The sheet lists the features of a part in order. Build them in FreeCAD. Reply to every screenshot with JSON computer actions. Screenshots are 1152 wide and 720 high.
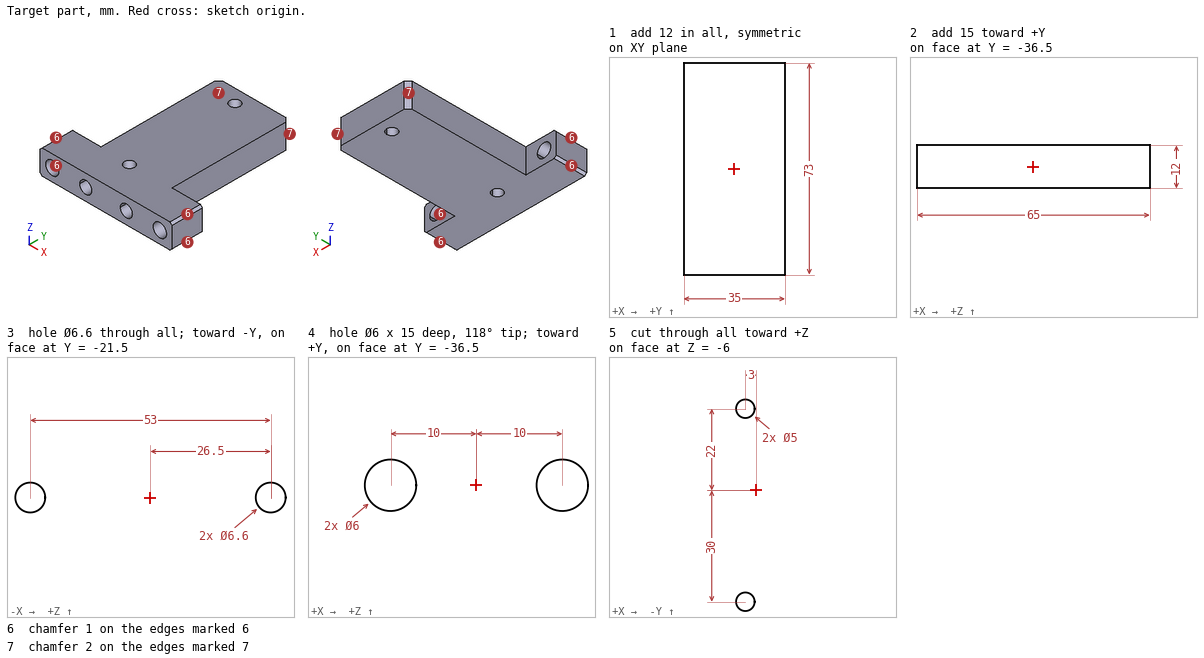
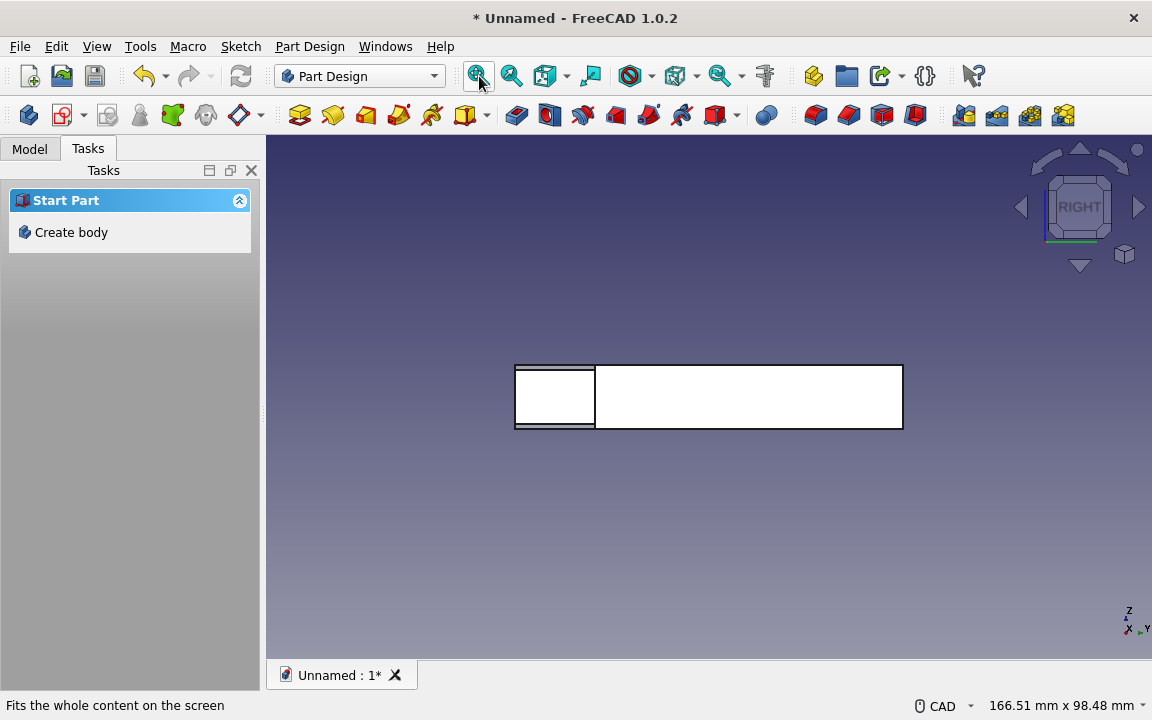
{"action": "left_click", "coordinate": [903, 396]}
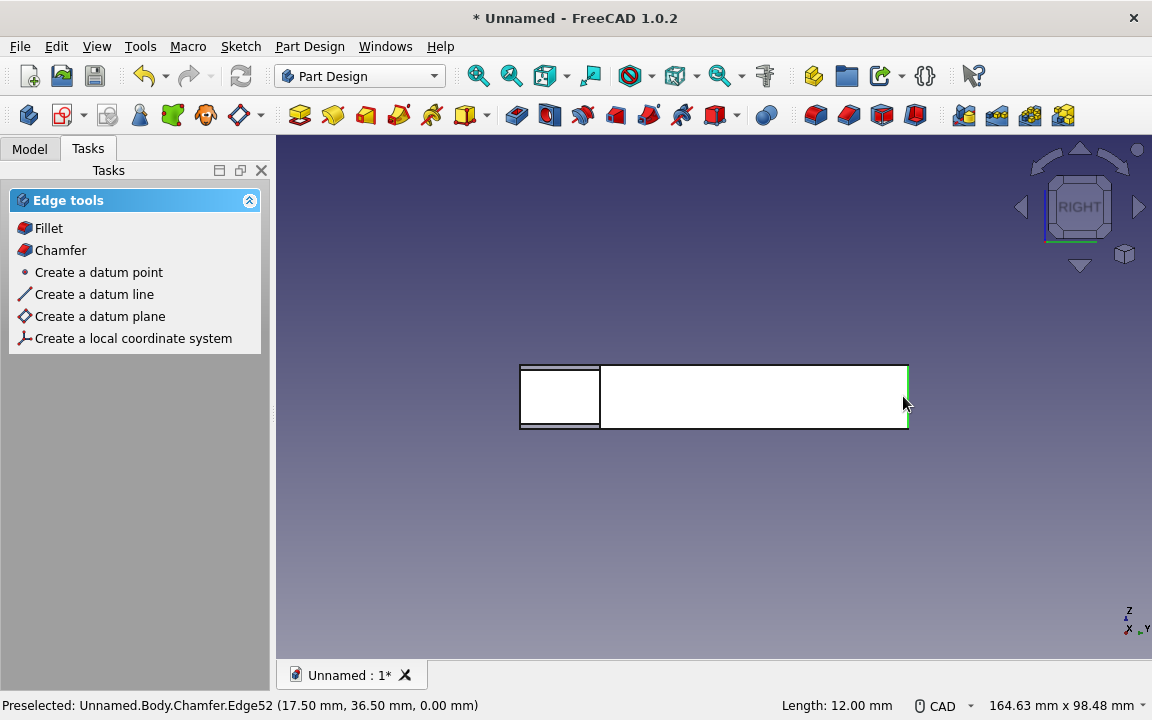
{"action": "key", "text": "5"}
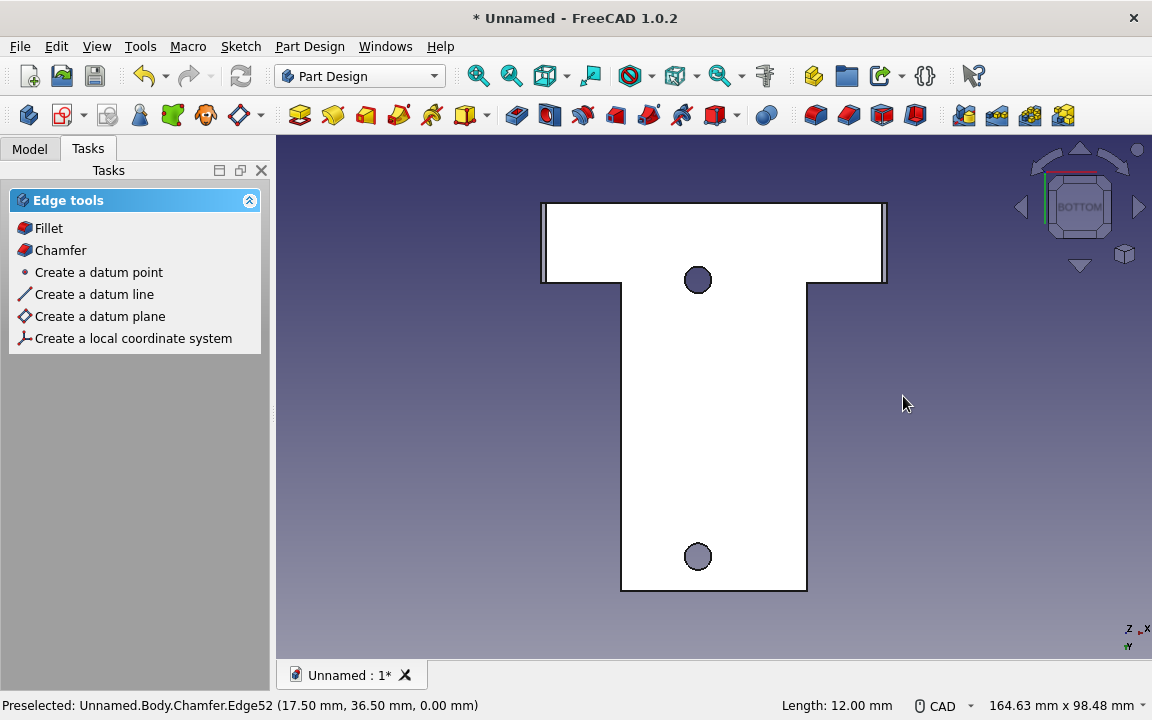
{"action": "key", "text": "4"}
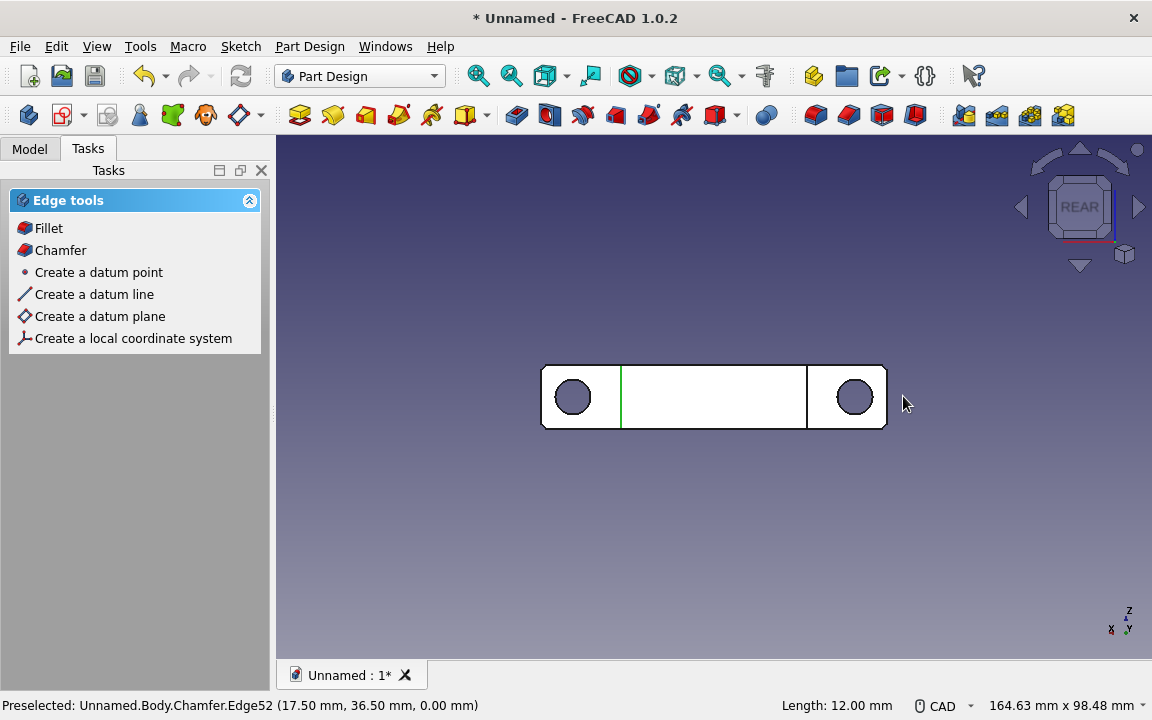
{"action": "left_click", "coordinate": [479, 76]}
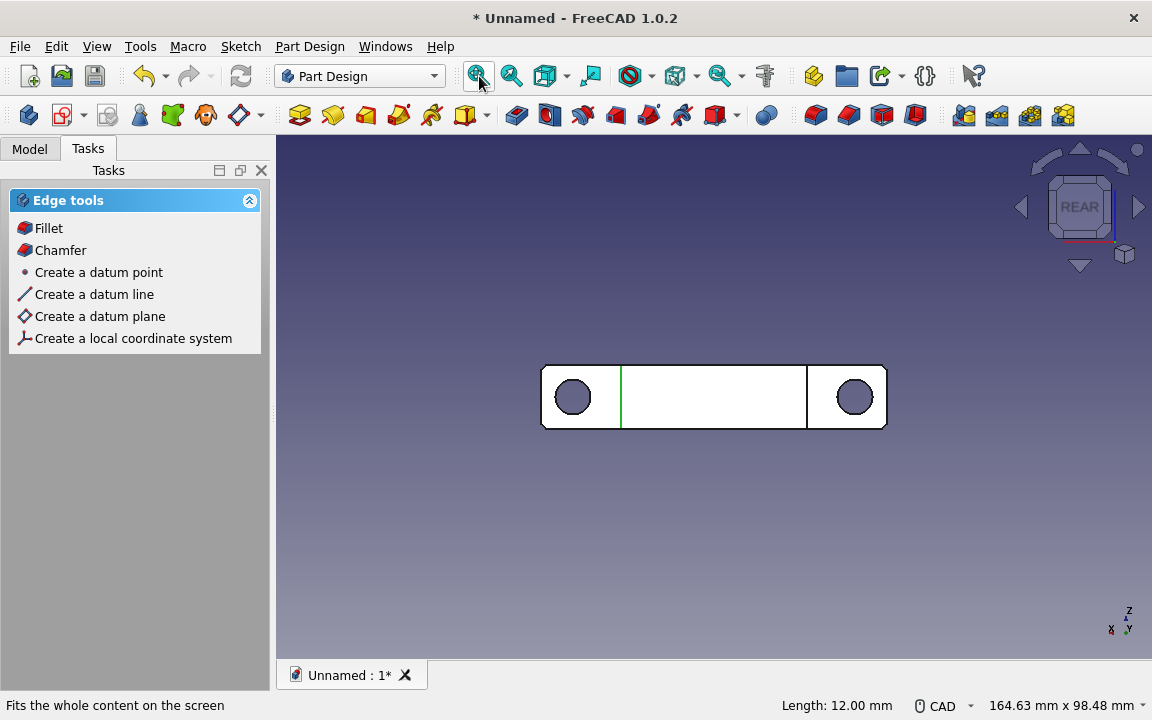
{"action": "left_click", "coordinate": [807, 396], "text": "ctrl"}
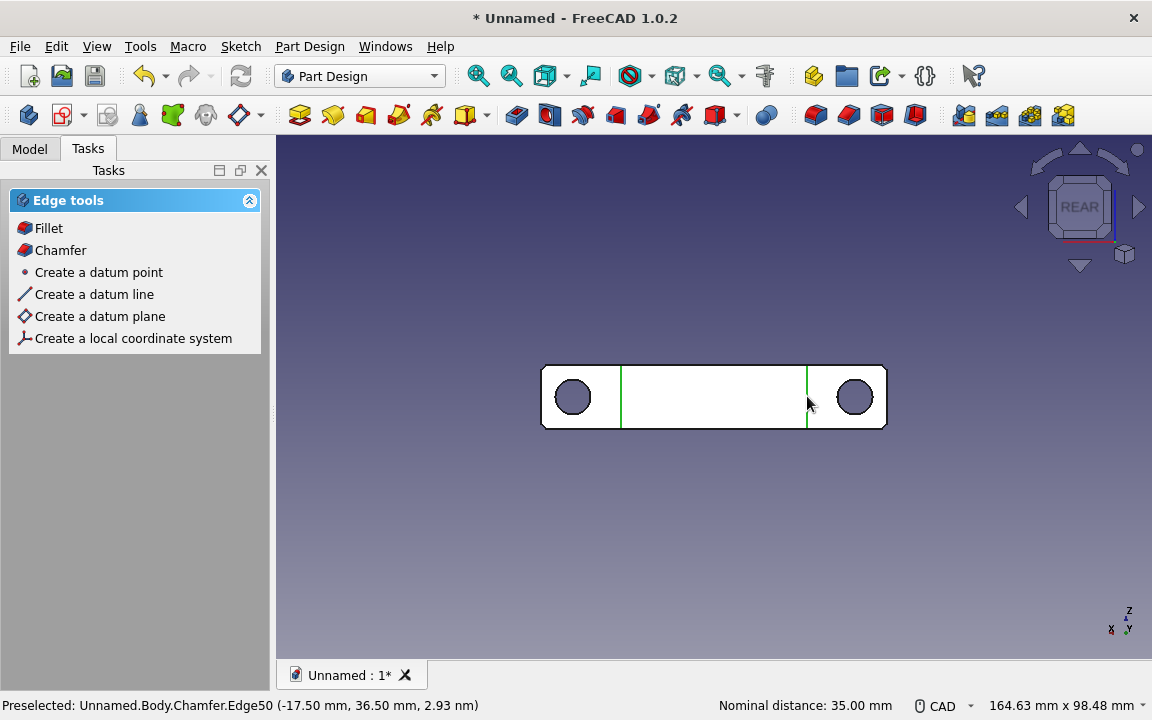
{"action": "left_click", "coordinate": [849, 116]}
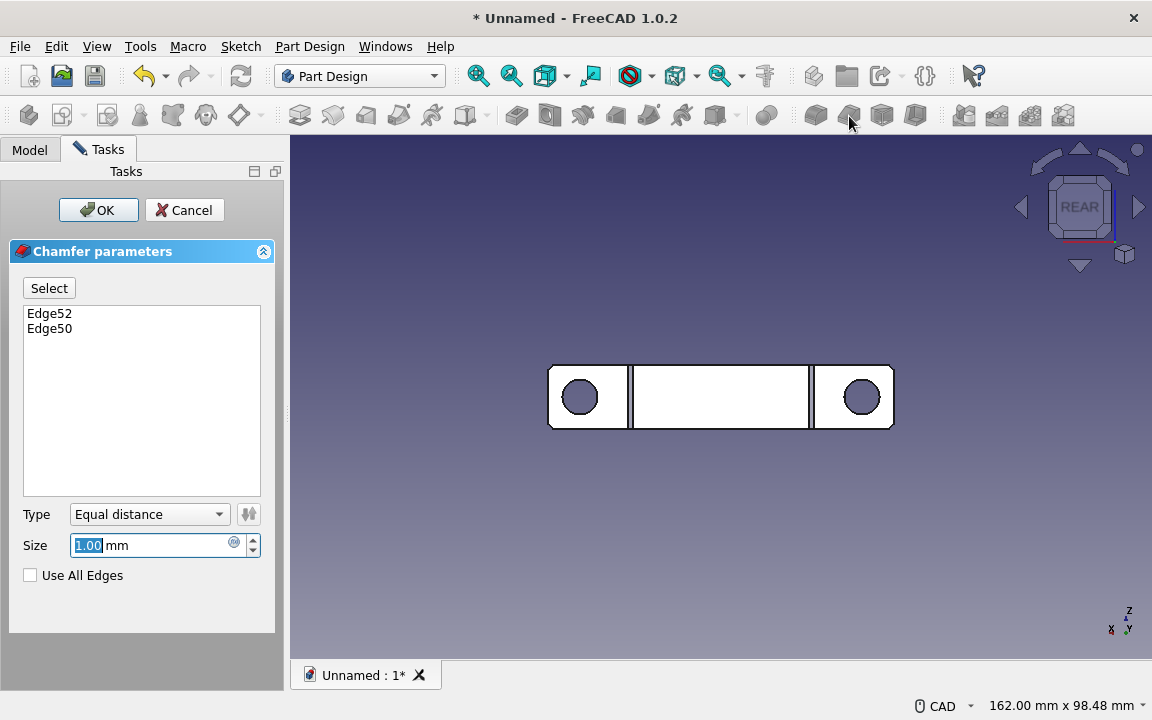
{"action": "type", "text": "2"}
{"action": "key", "text": "Tab"}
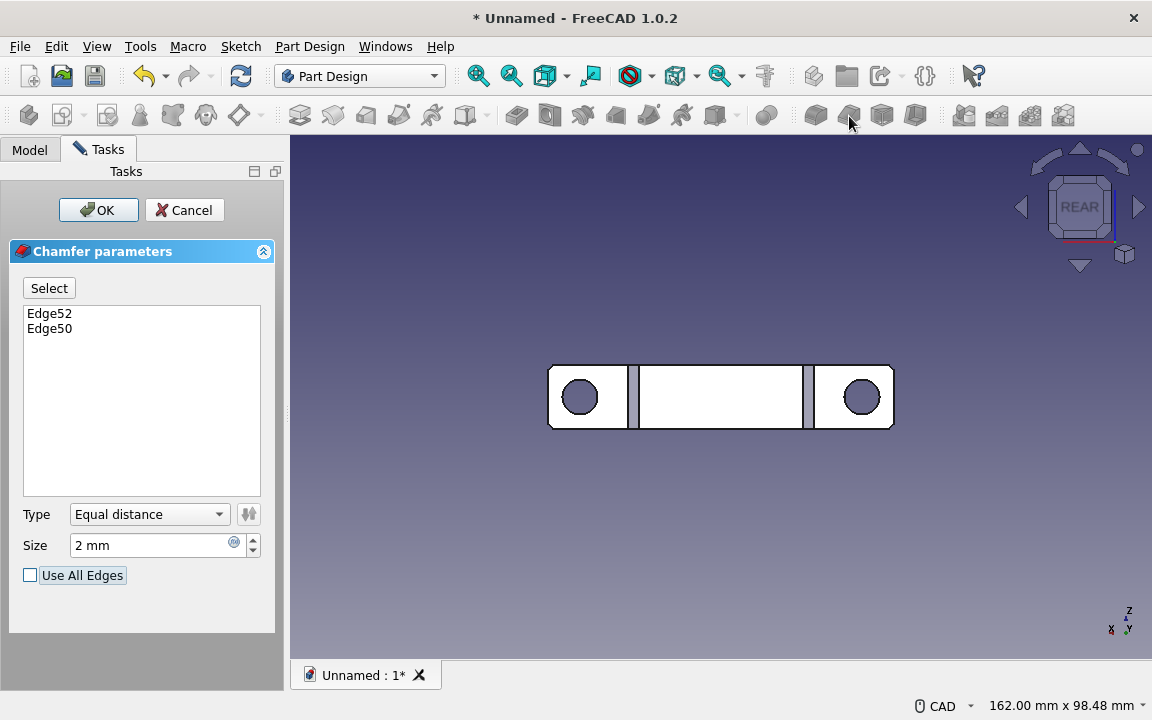
{"action": "left_click", "coordinate": [99, 210]}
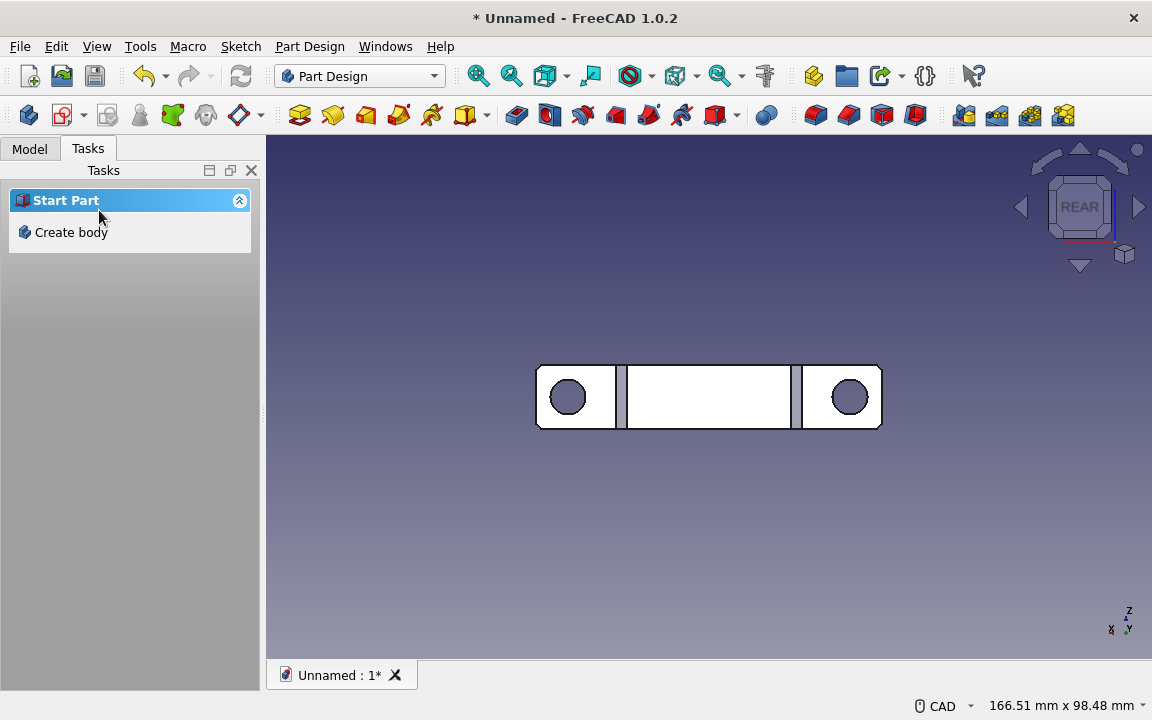
{"action": "key", "text": "0"}